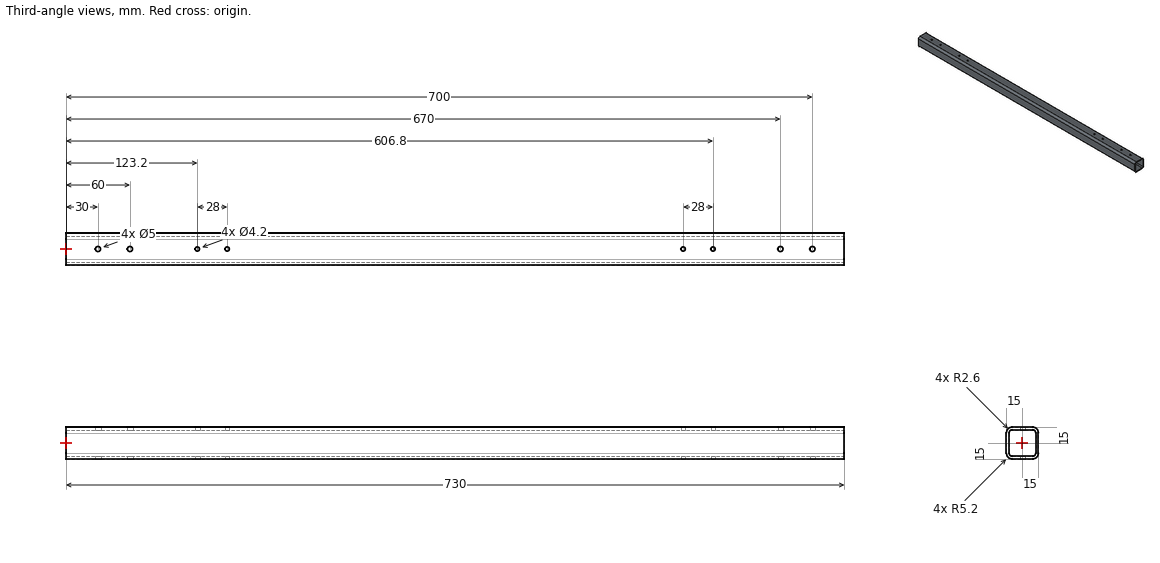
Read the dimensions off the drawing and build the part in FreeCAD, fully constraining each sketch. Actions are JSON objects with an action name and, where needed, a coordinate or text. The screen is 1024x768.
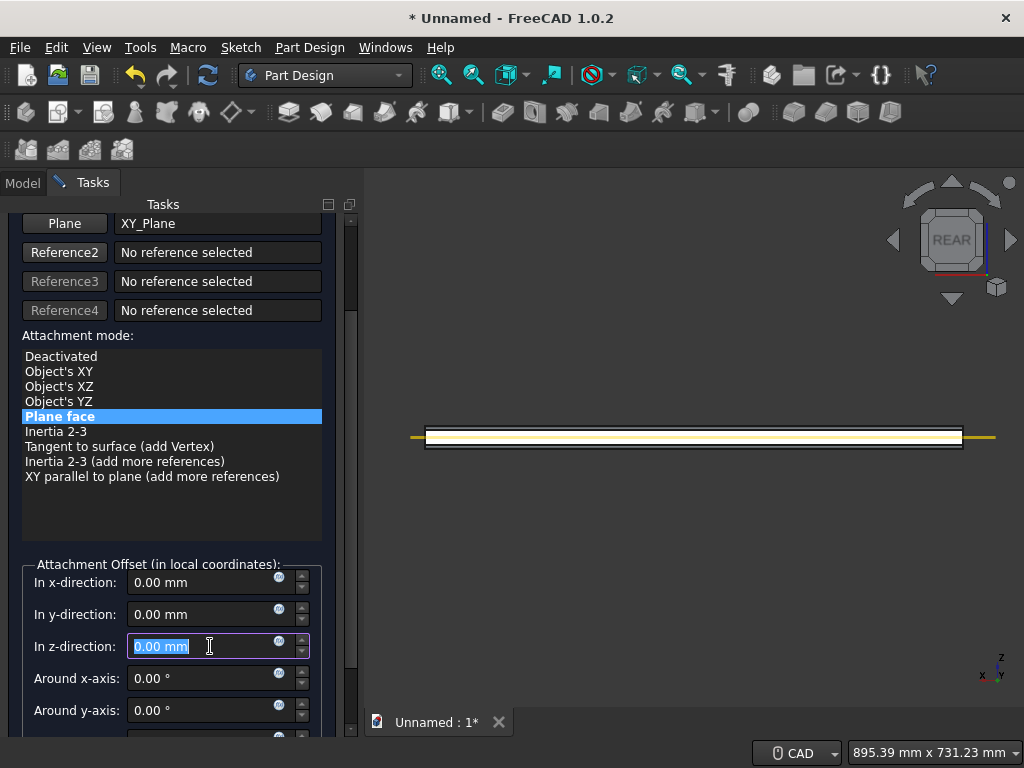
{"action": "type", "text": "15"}
{"action": "key", "text": "Tab"}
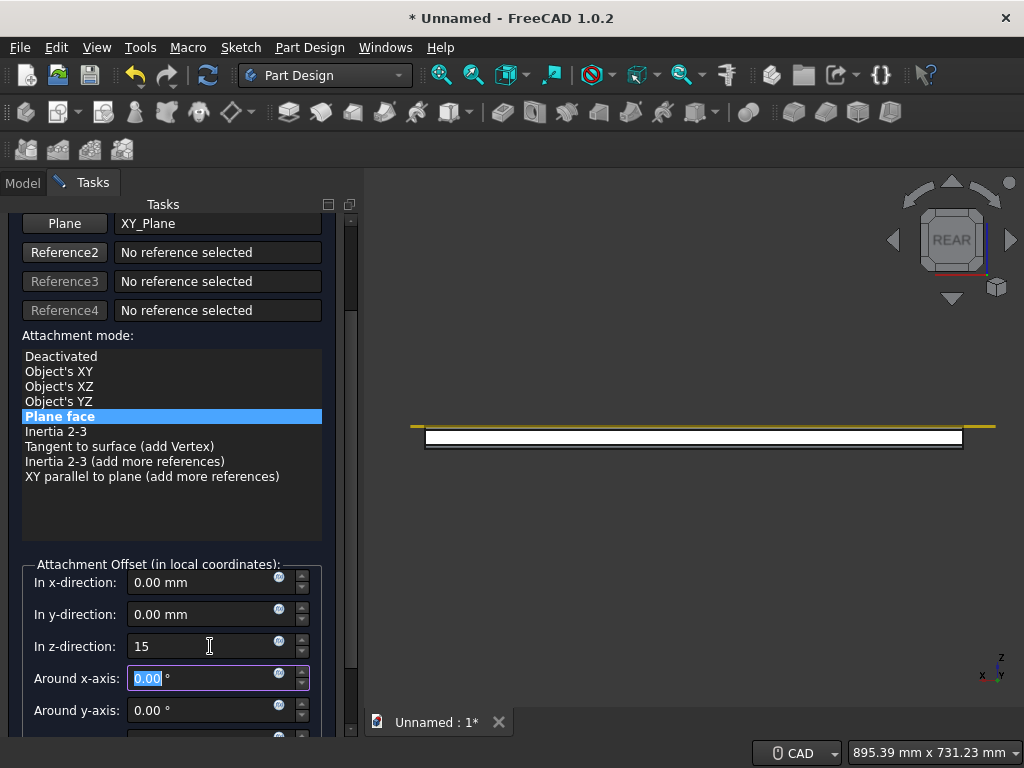
{"action": "scroll", "coordinate": [351, 475], "scroll_direction": "up", "scroll_amount": 3}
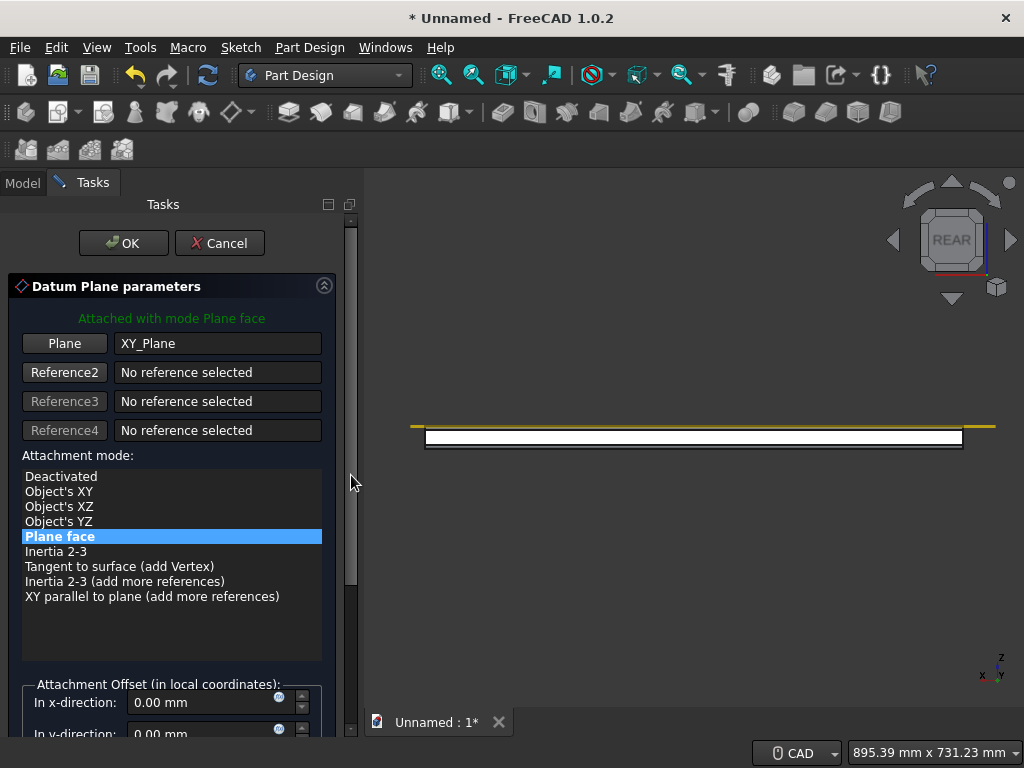
{"action": "left_click", "coordinate": [124, 243]}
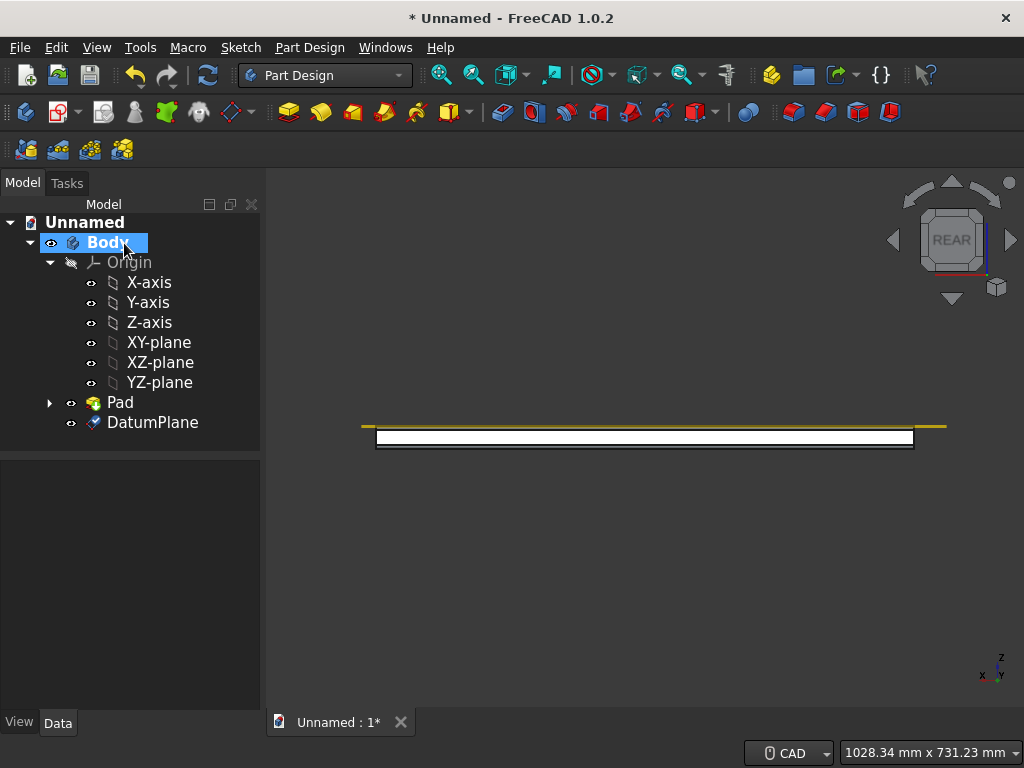
{"action": "left_click", "coordinate": [116, 423]}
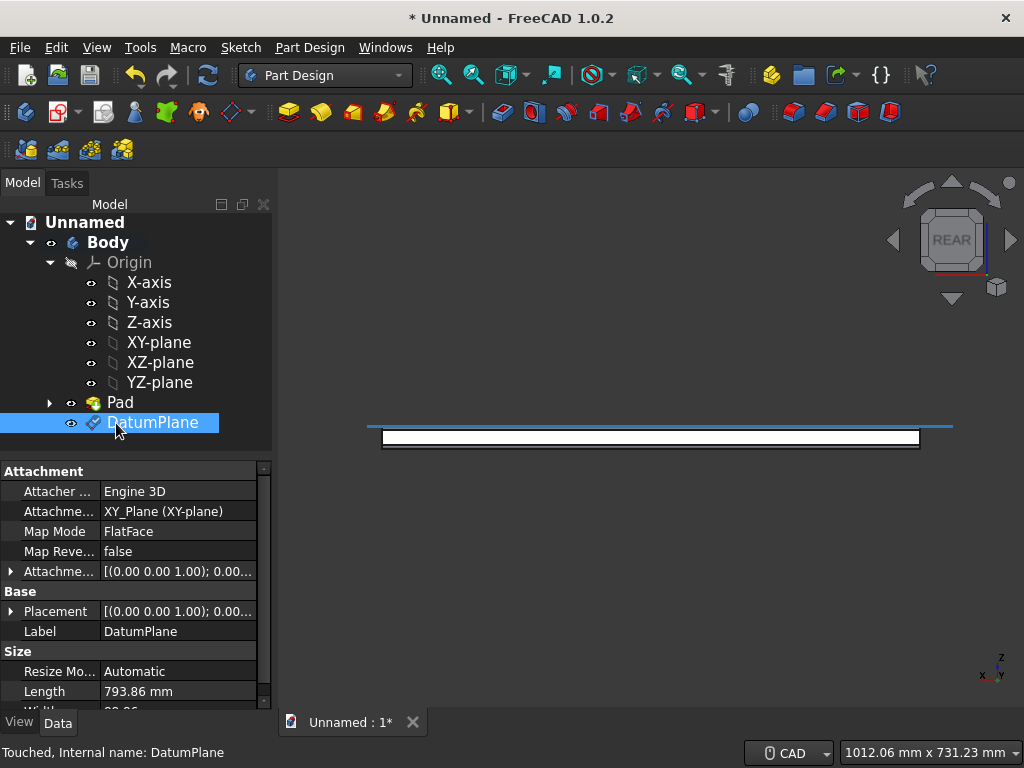
{"action": "left_click", "coordinate": [58, 112]}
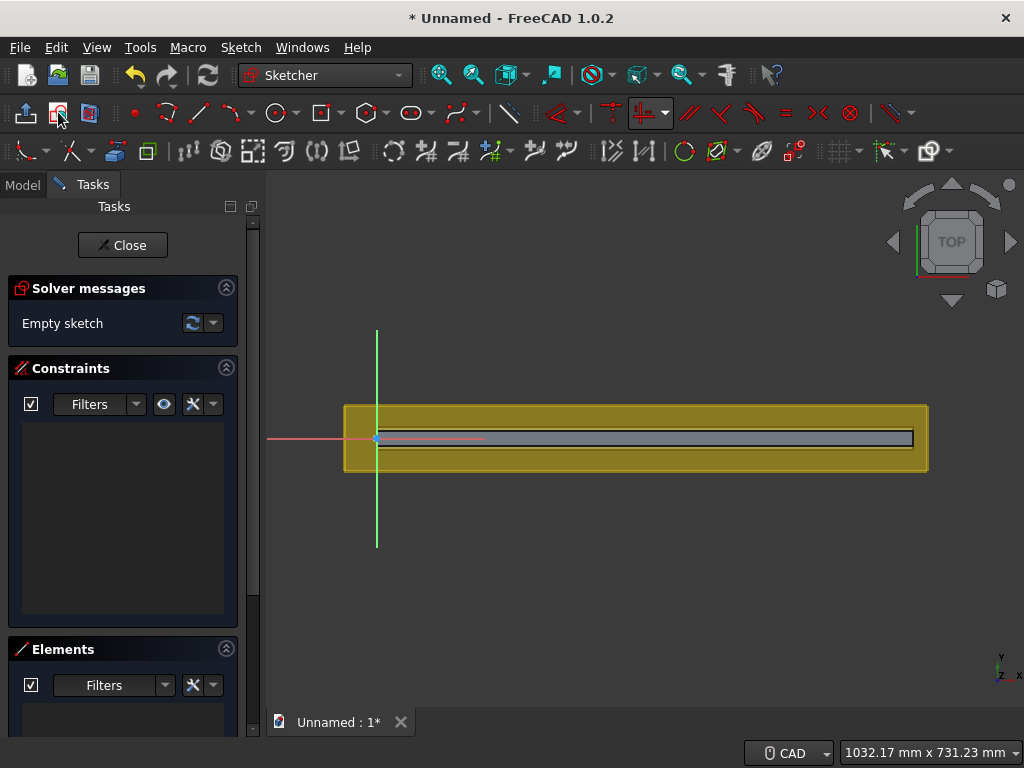
{"action": "left_click", "coordinate": [276, 114]}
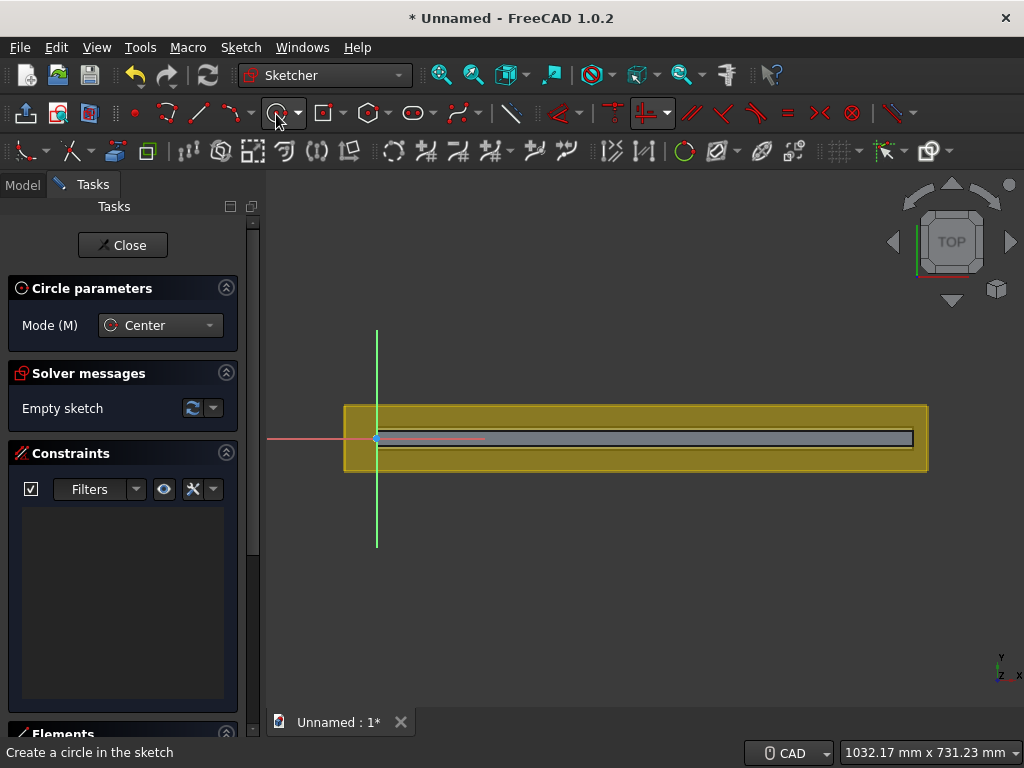
{"action": "scroll", "coordinate": [467, 439], "scroll_direction": "up", "scroll_amount": 14}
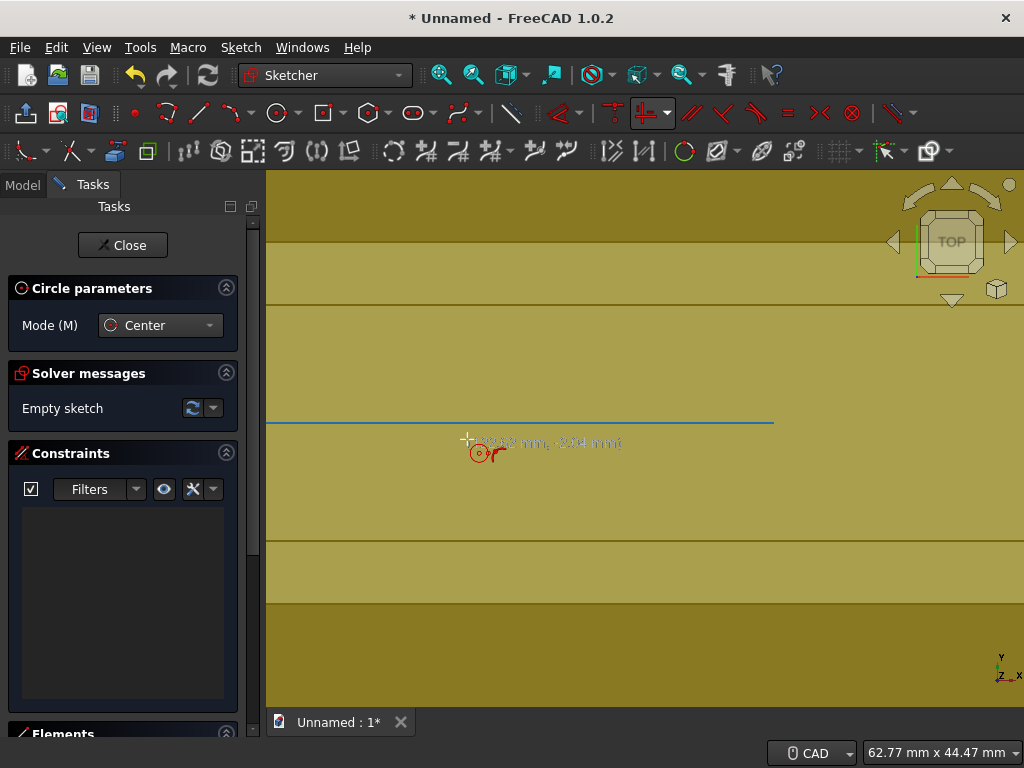
{"action": "scroll", "coordinate": [467, 439], "scroll_direction": "down", "scroll_amount": 15}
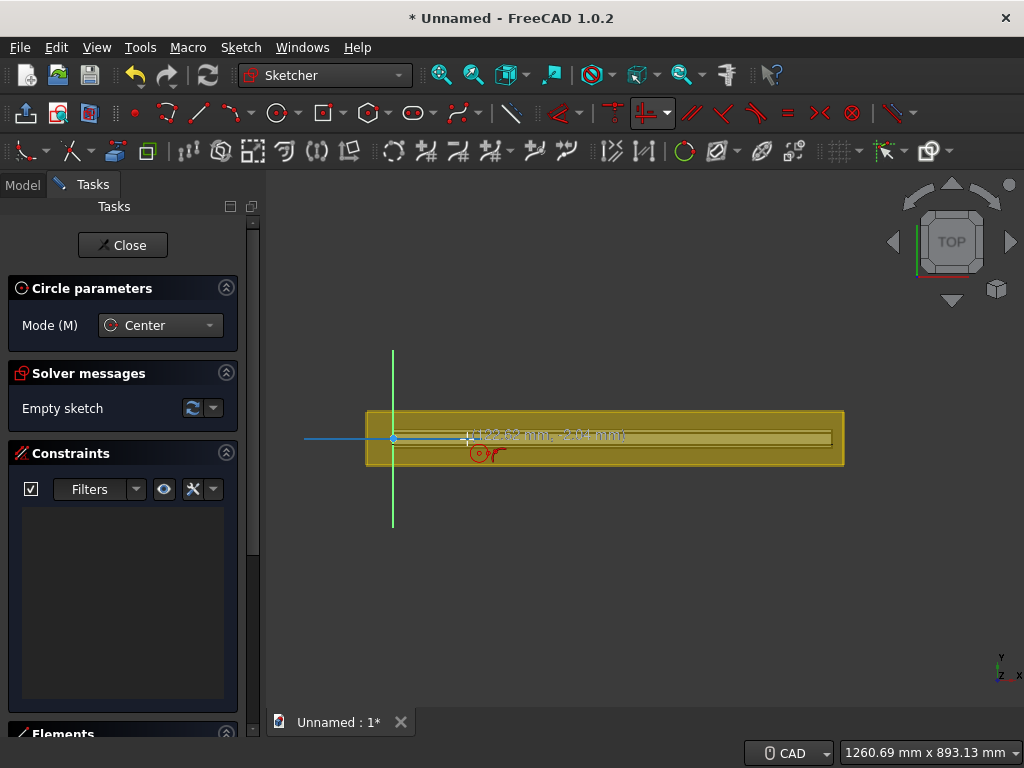
{"action": "left_click", "coordinate": [467, 439]}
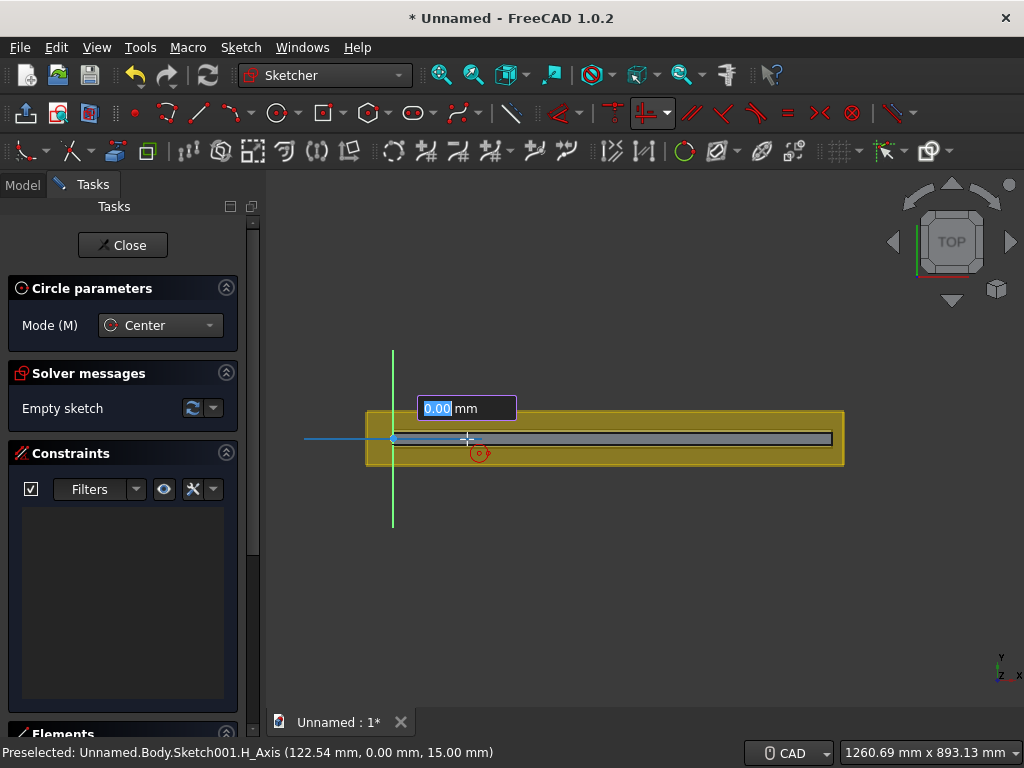
{"action": "scroll", "coordinate": [468, 437], "scroll_direction": "up", "scroll_amount": 13}
{"action": "mouse_move", "coordinate": [462, 437]}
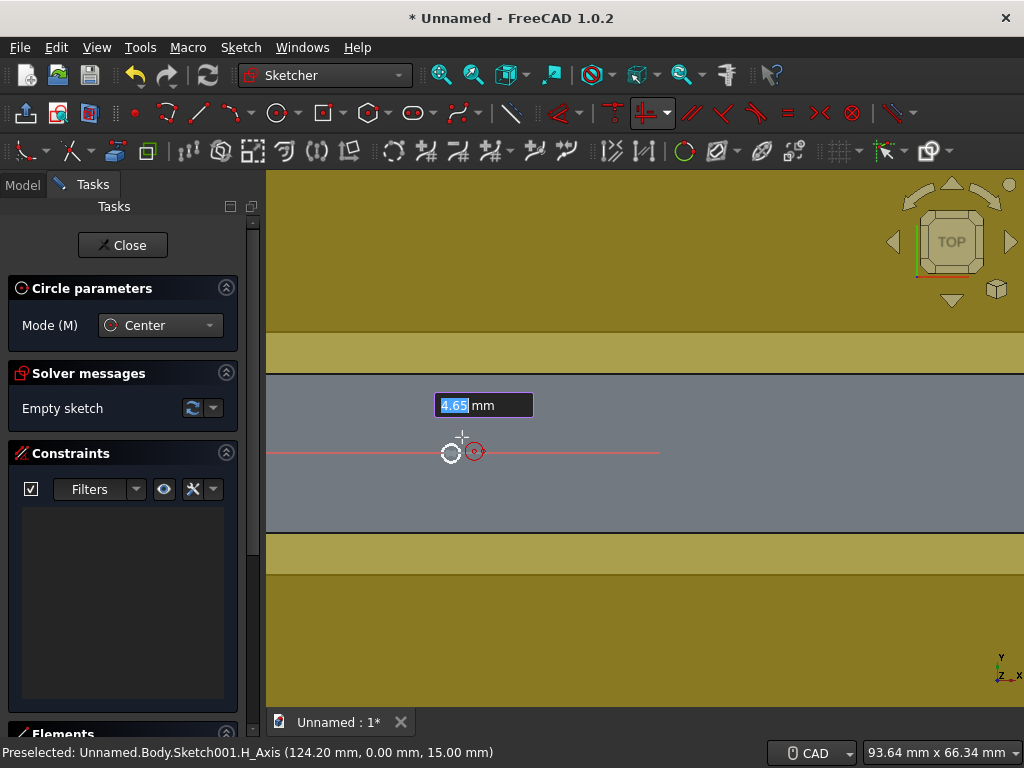
{"action": "type", "text": "4.2"}
{"action": "key", "text": "Return"}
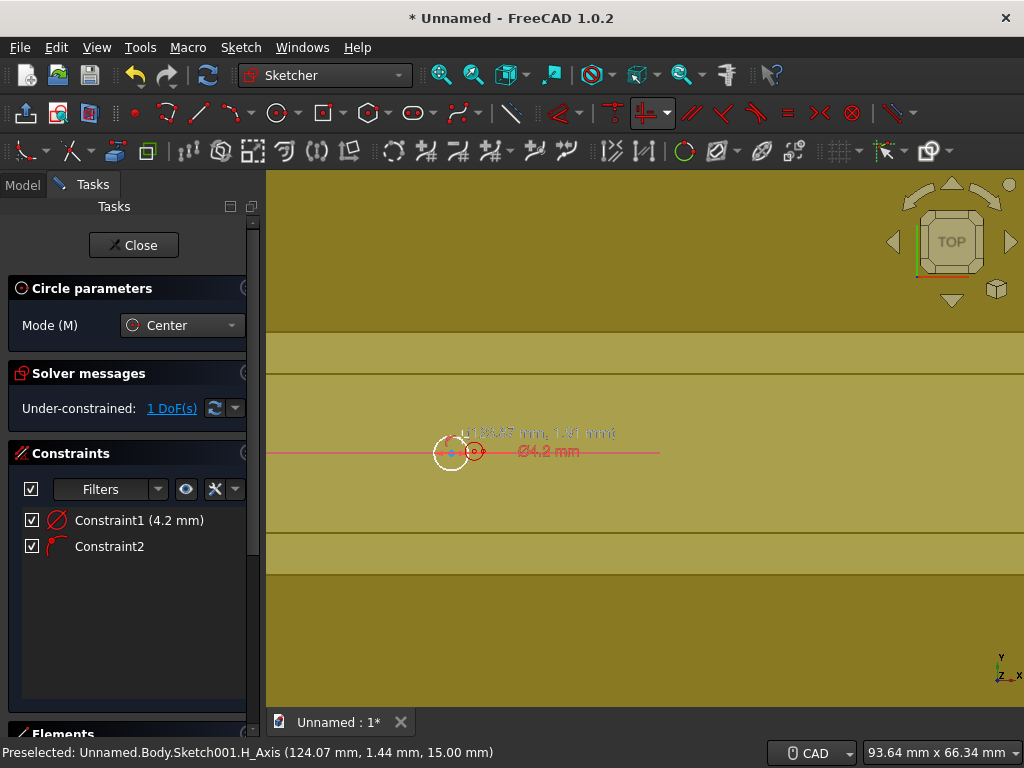
{"action": "scroll", "coordinate": [683, 453], "scroll_direction": "up", "scroll_amount": 2}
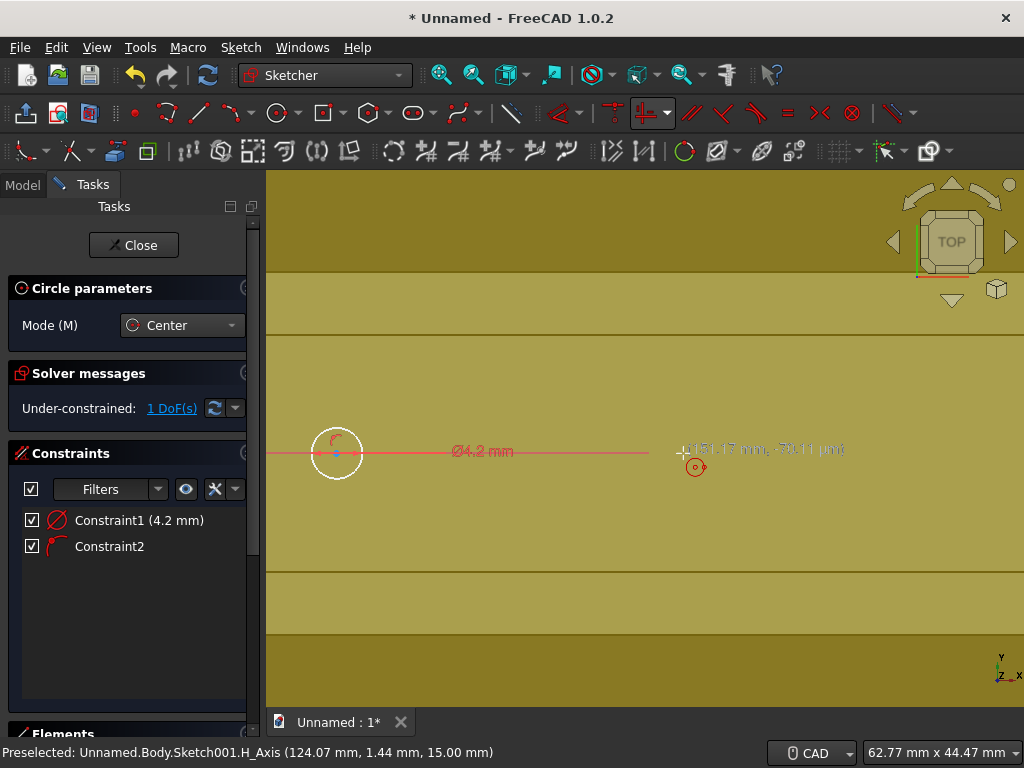
{"action": "scroll", "coordinate": [474, 438], "scroll_direction": "down", "scroll_amount": 15}